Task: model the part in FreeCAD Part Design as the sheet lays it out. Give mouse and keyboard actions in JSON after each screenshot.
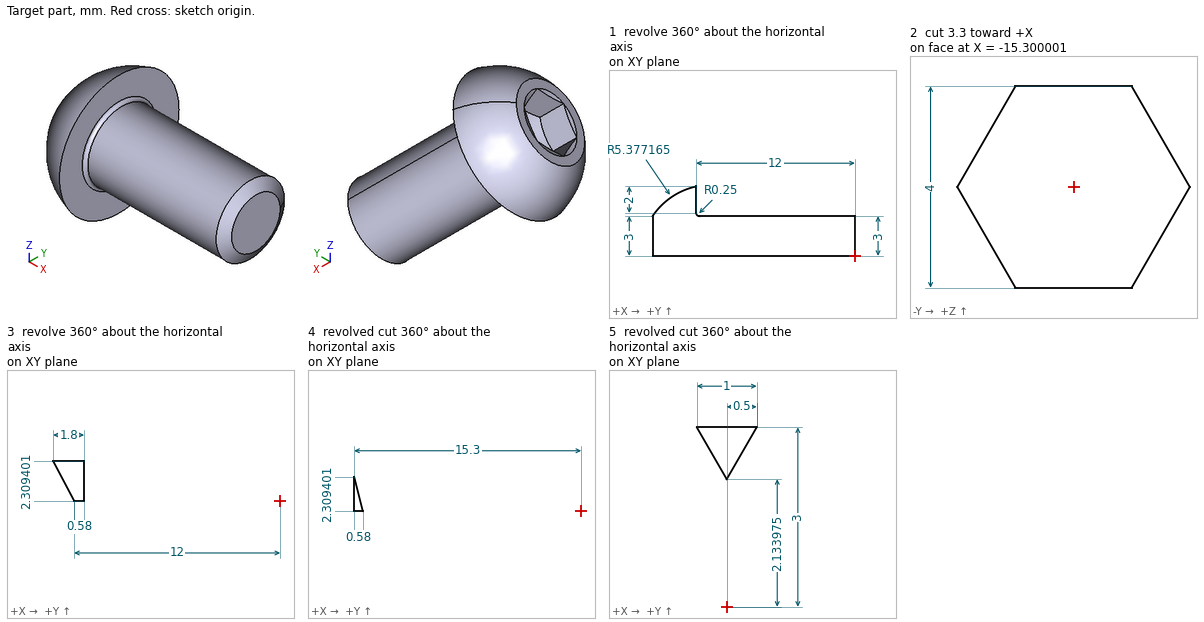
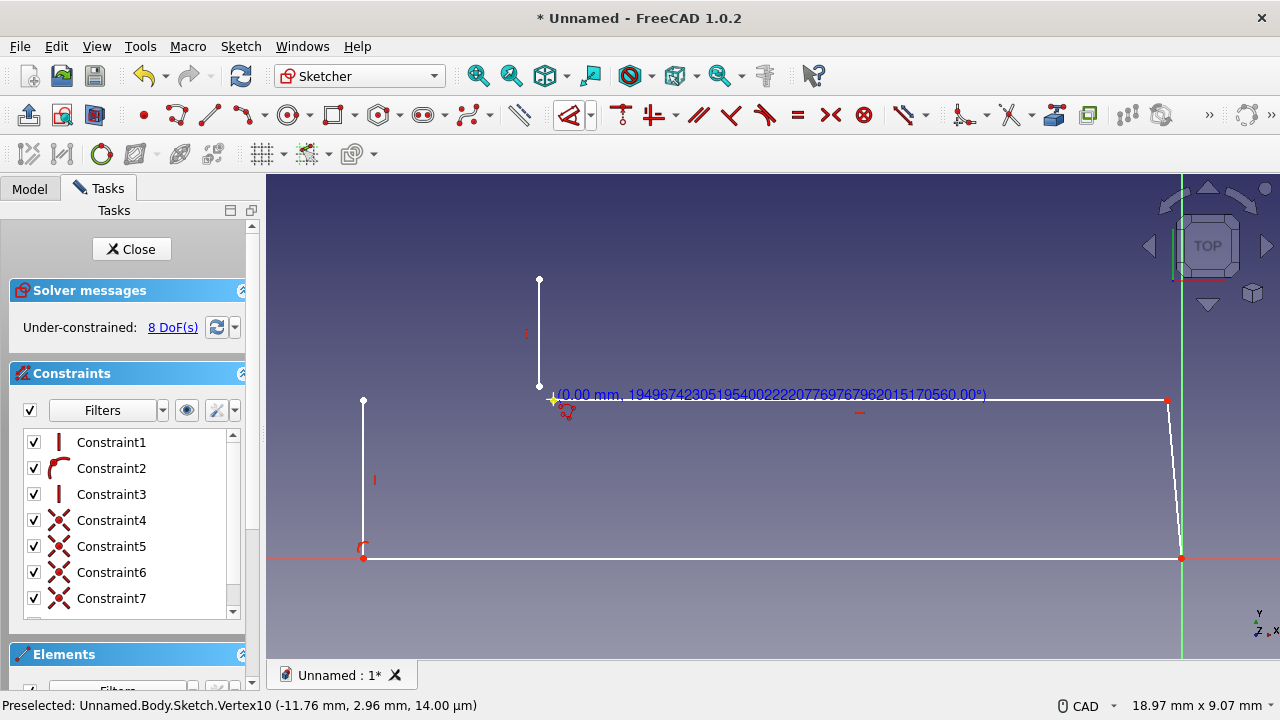
{"action": "left_click", "coordinate": [242, 116]}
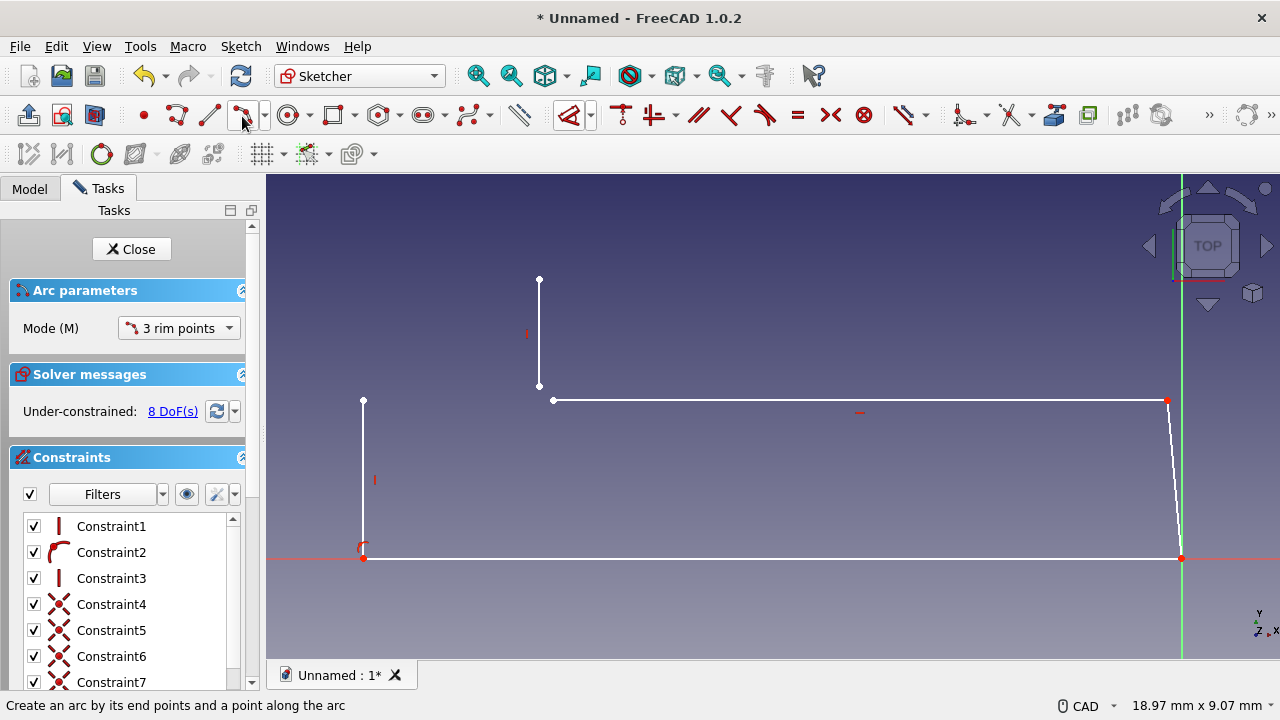
{"action": "left_click", "coordinate": [539, 279]}
{"action": "left_click", "coordinate": [363, 400]}
{"action": "left_click", "coordinate": [440, 321]}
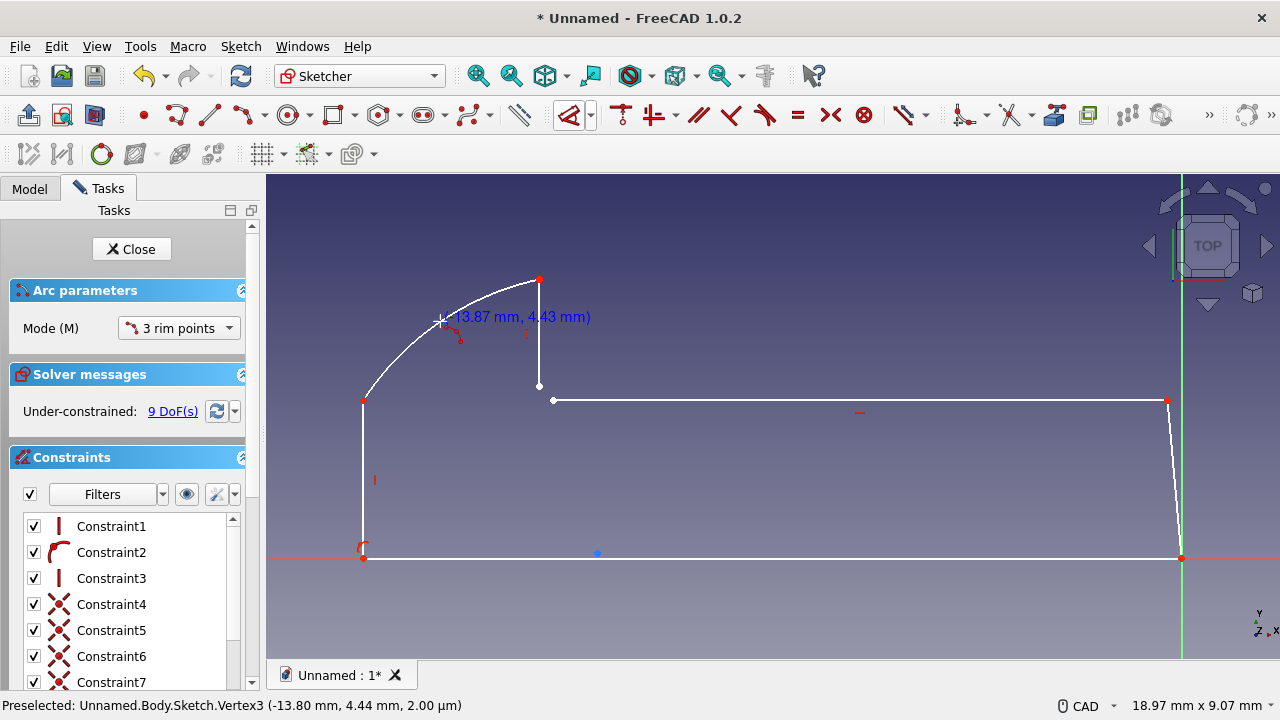
{"action": "left_click", "coordinate": [553, 400]}
{"action": "left_click", "coordinate": [539, 387]}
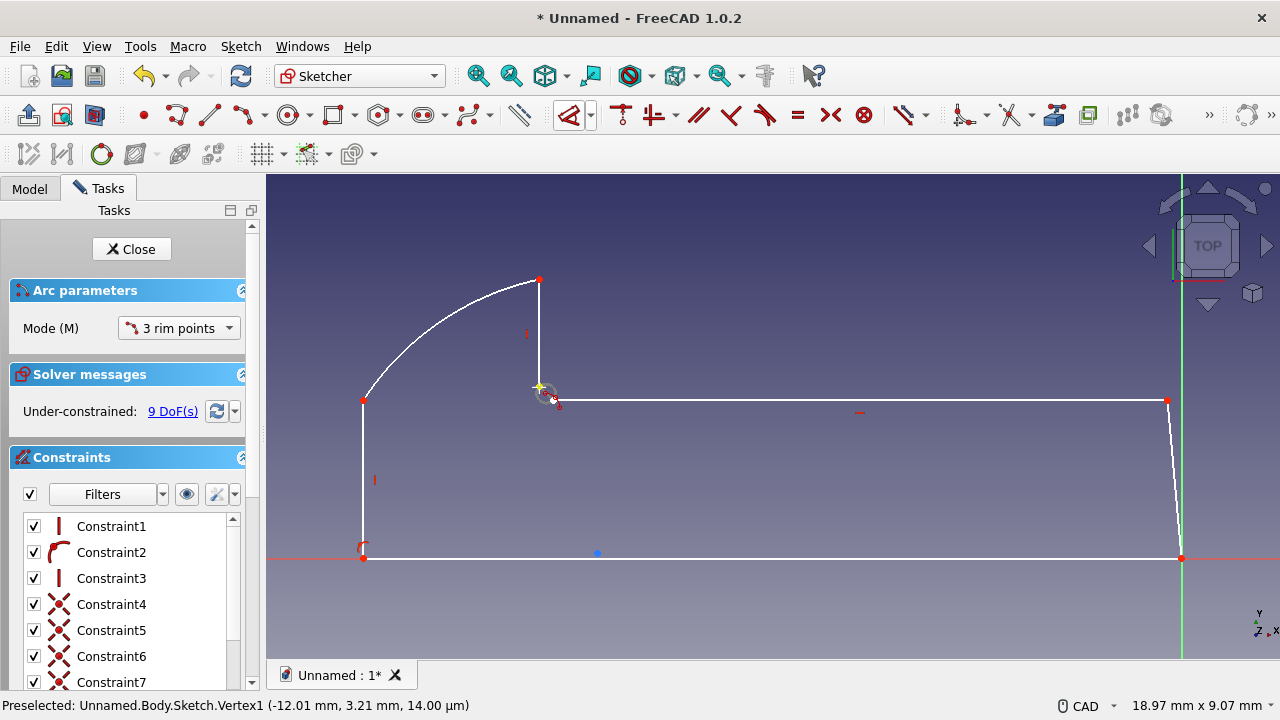
{"action": "scroll", "coordinate": [544, 394], "scroll_direction": "up", "scroll_amount": 8}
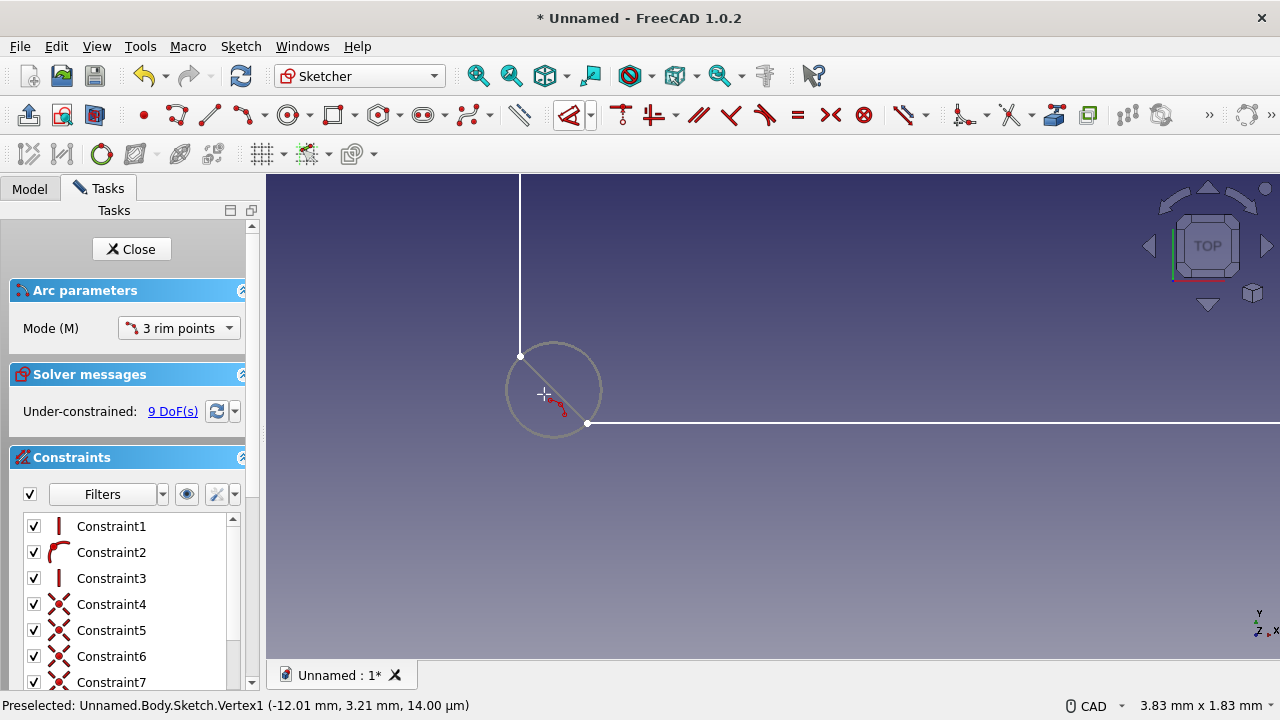
{"action": "left_click", "coordinate": [543, 394]}
{"action": "key", "text": "Escape"}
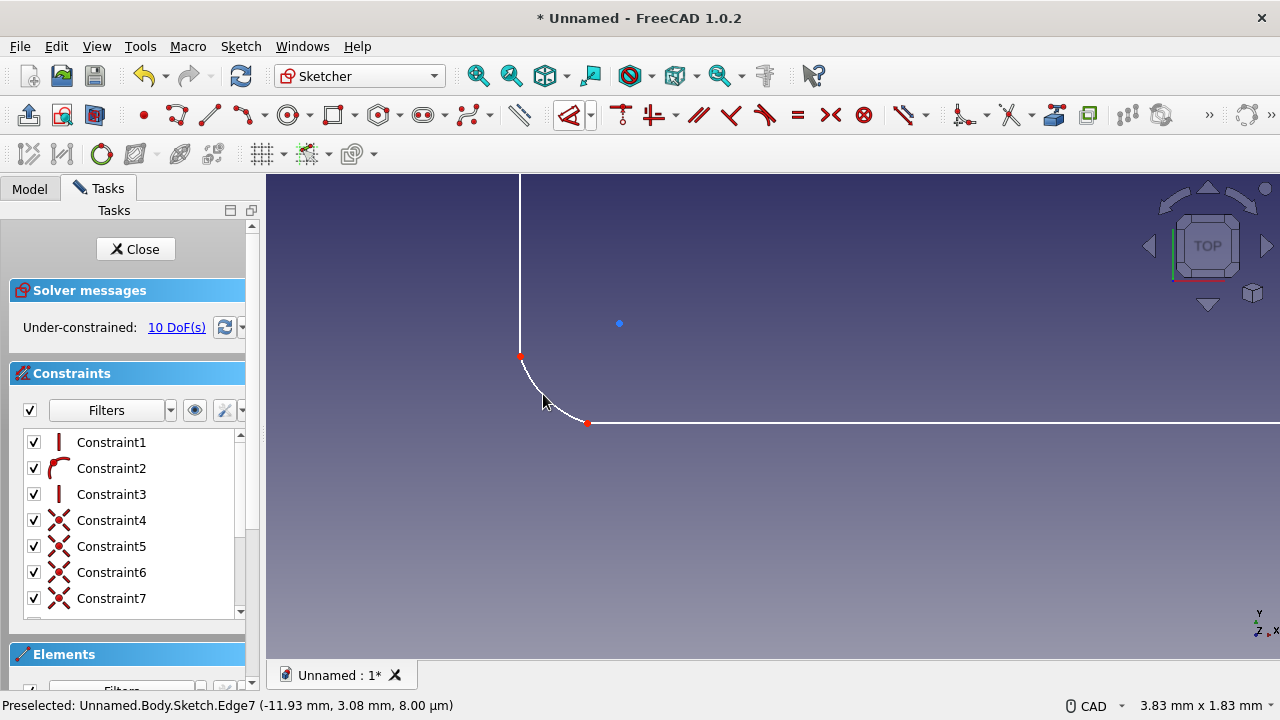
{"action": "scroll", "coordinate": [553, 402], "scroll_direction": "down", "scroll_amount": 10}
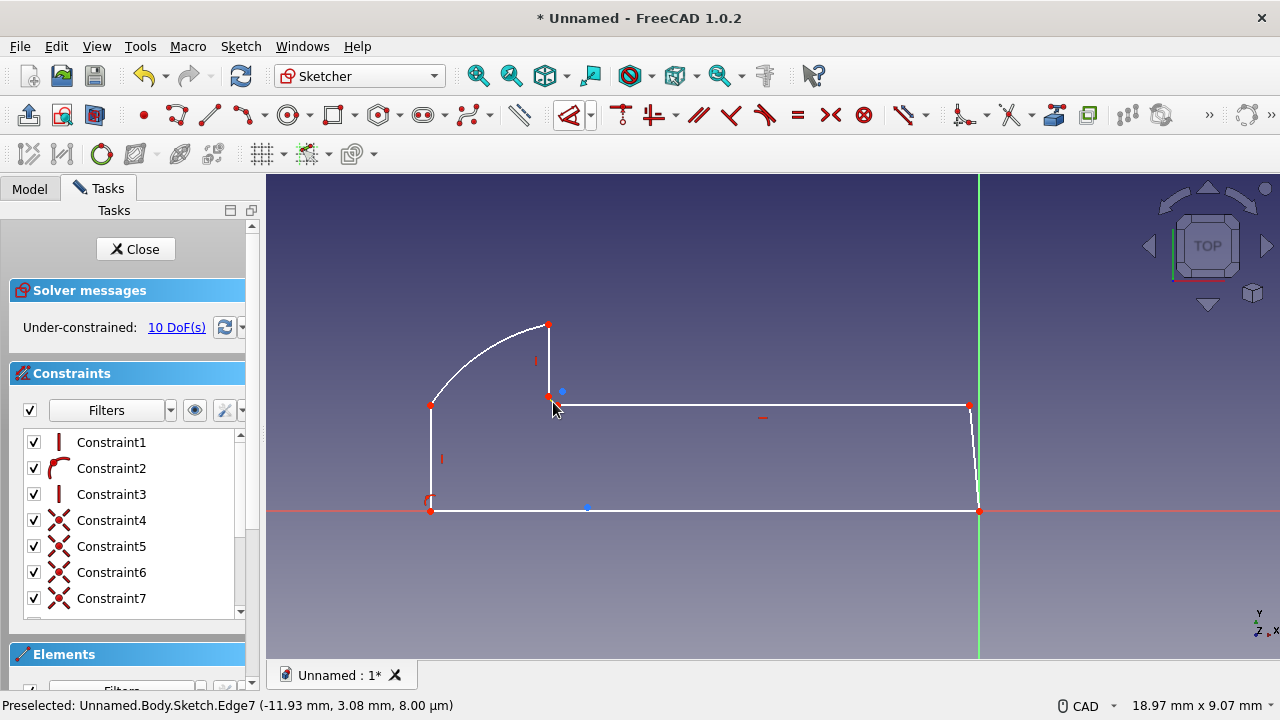
{"action": "left_click", "coordinate": [549, 382]}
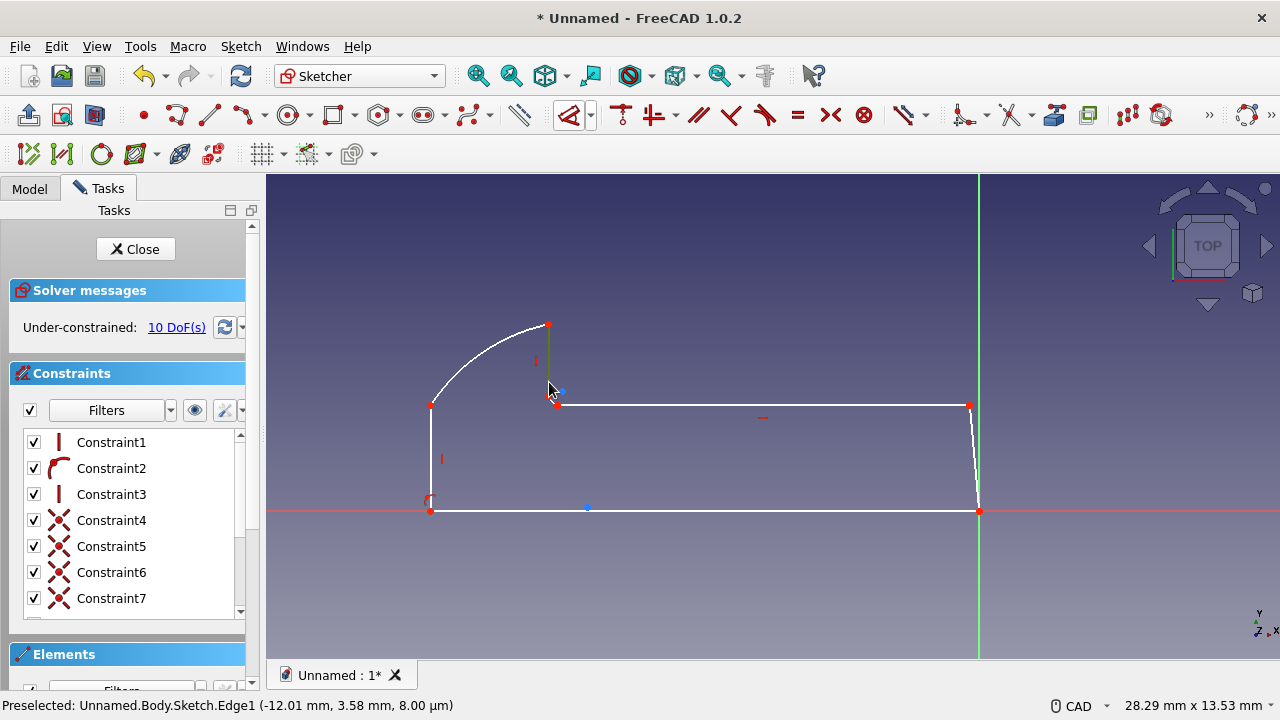
{"action": "scroll", "coordinate": [552, 402], "scroll_direction": "up", "scroll_amount": 4}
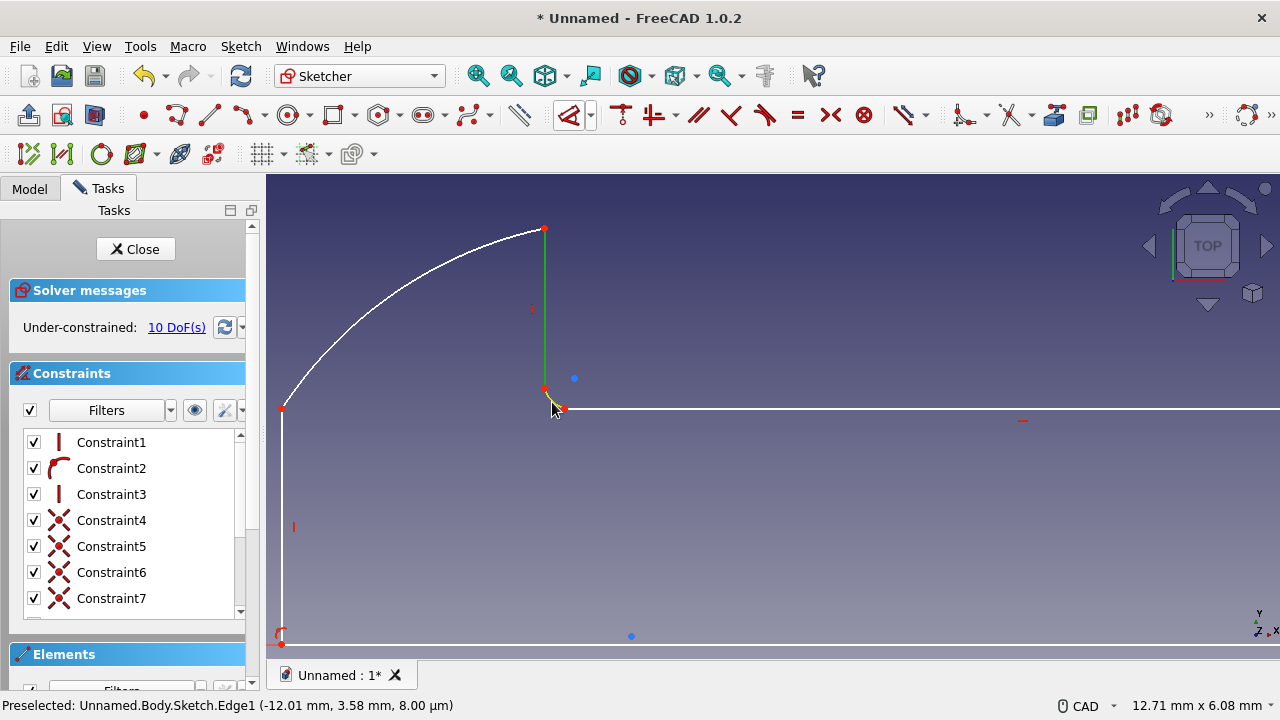
{"action": "left_click", "coordinate": [552, 401]}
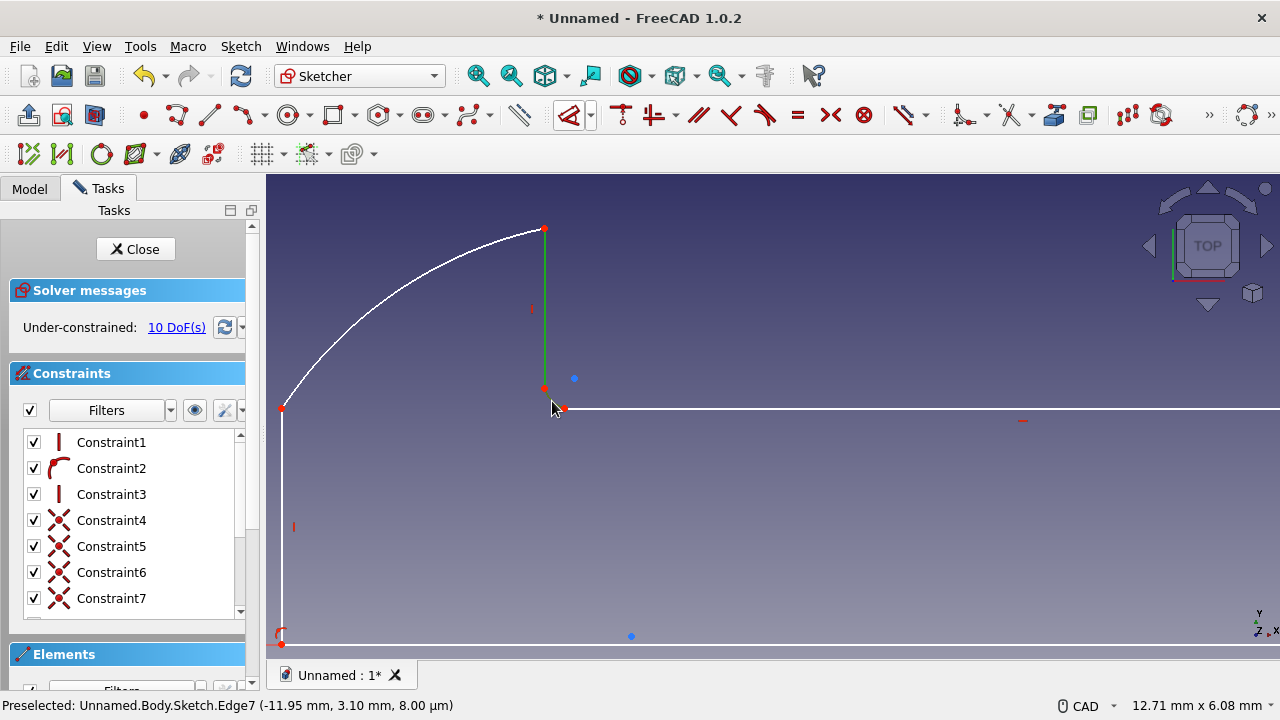
{"action": "left_click", "coordinate": [765, 116]}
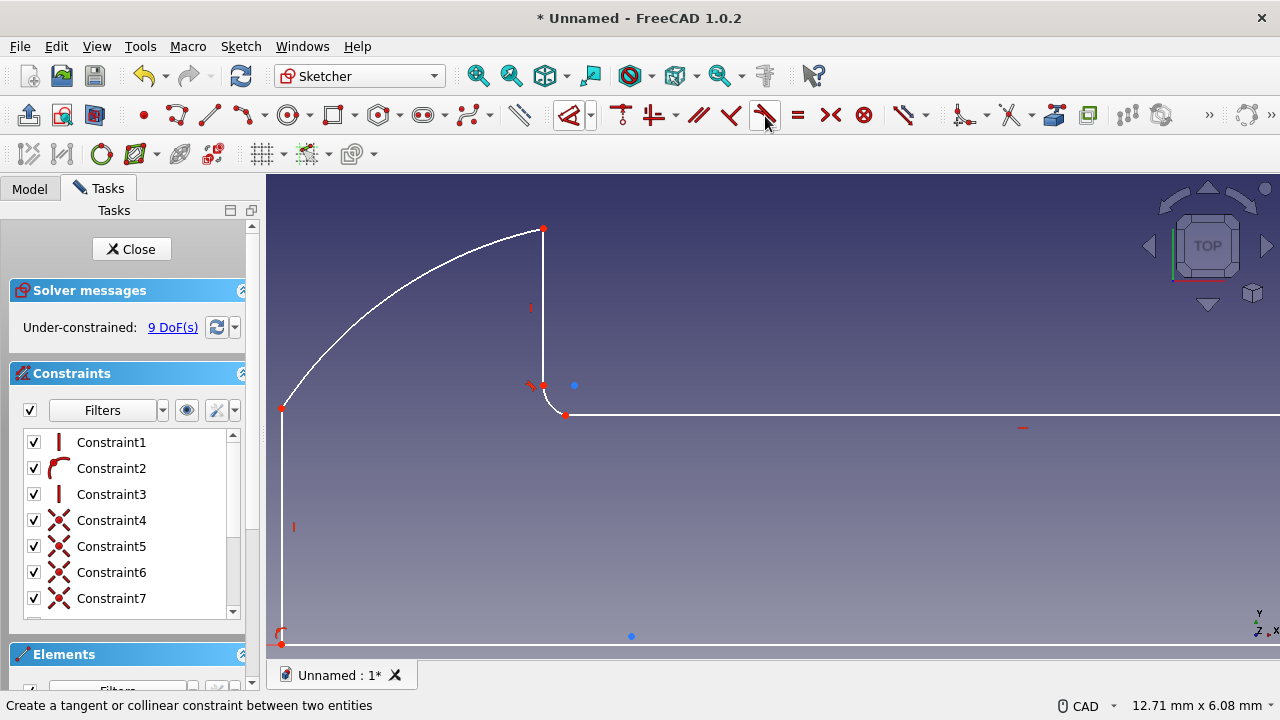
{"action": "left_click", "coordinate": [840, 415]}